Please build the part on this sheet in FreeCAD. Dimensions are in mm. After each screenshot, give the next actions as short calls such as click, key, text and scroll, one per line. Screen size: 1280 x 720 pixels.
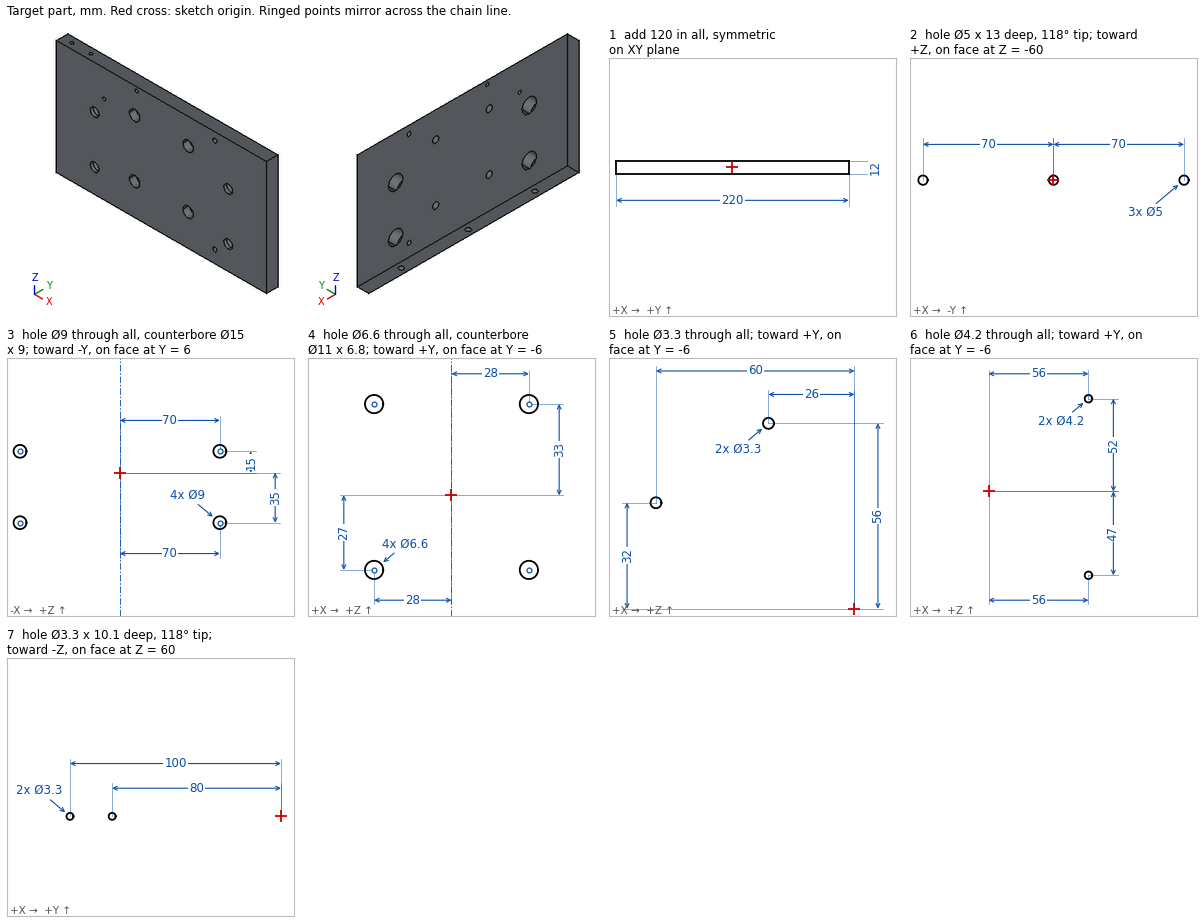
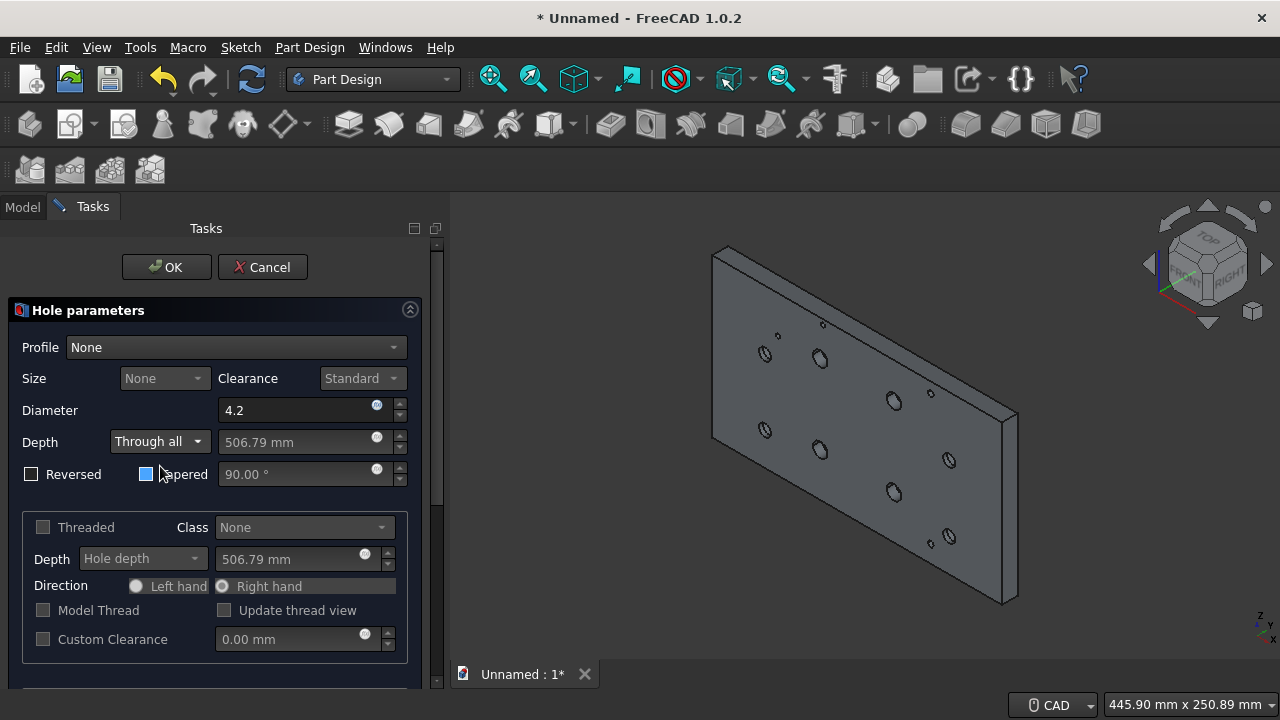
click(167, 267)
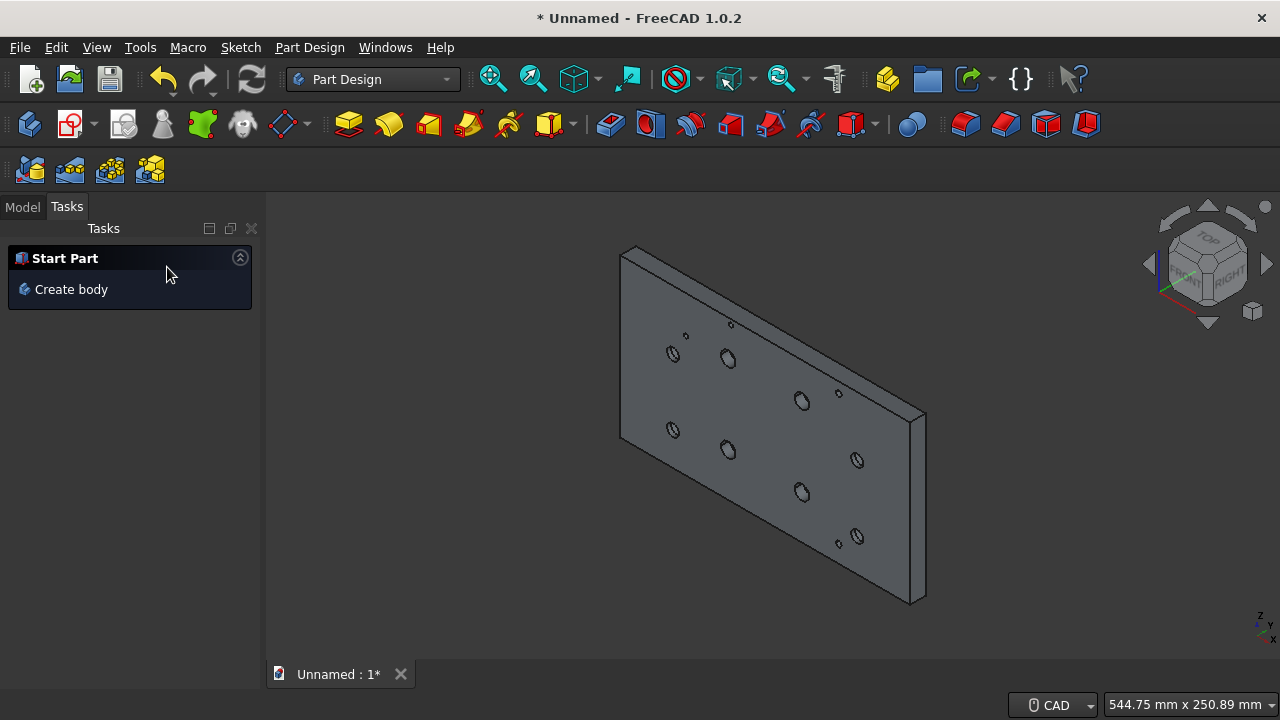
click(899, 404)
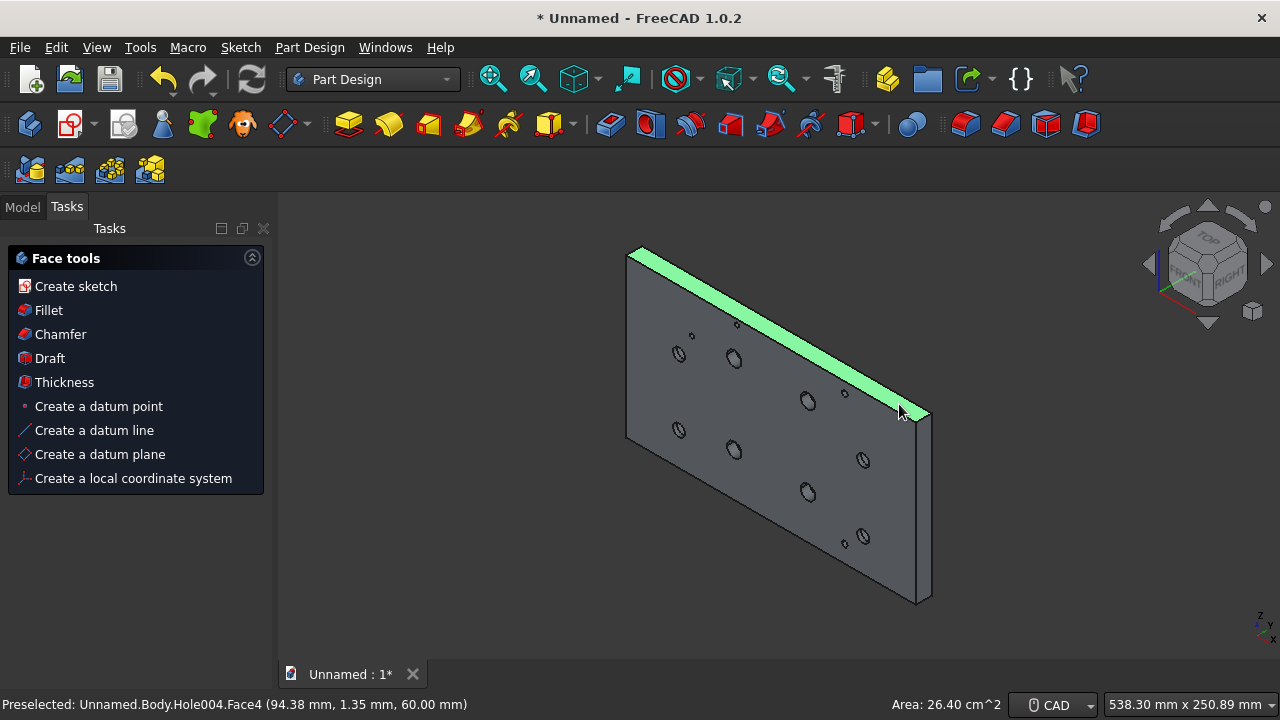
click(70, 124)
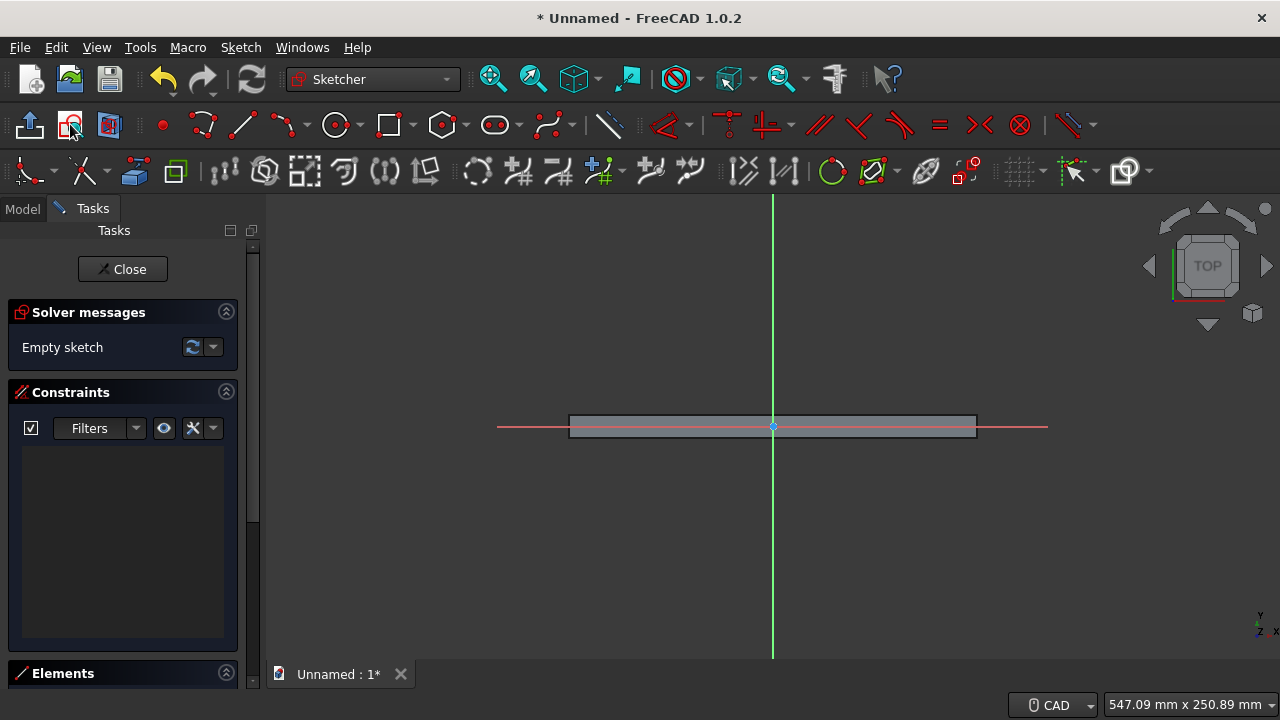
scroll(598, 426, up, 13)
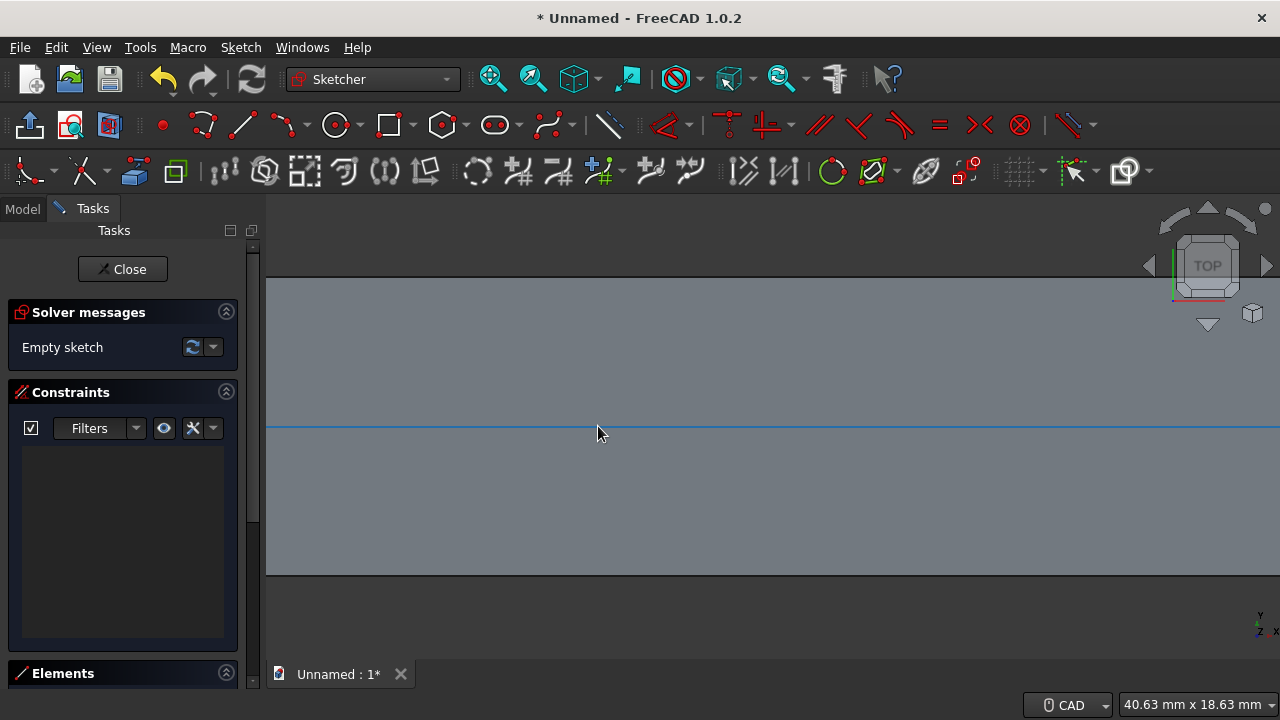
click(336, 126)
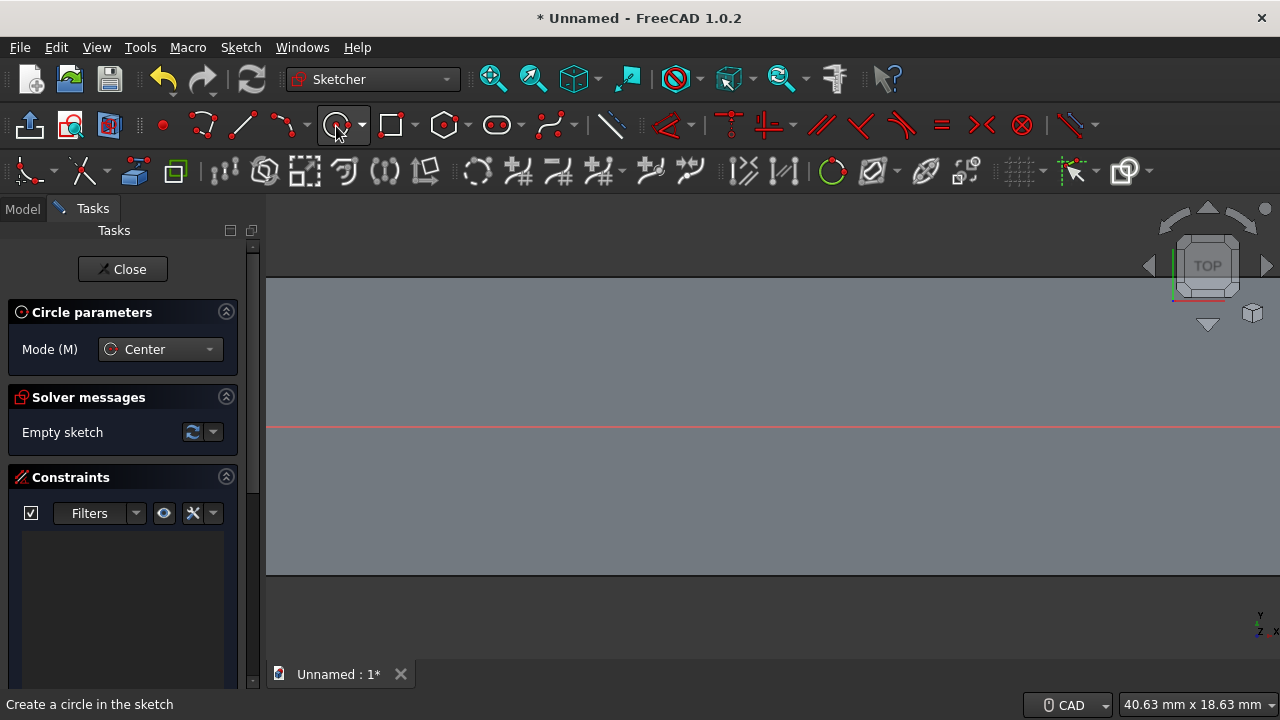
click(455, 426)
move(484, 397)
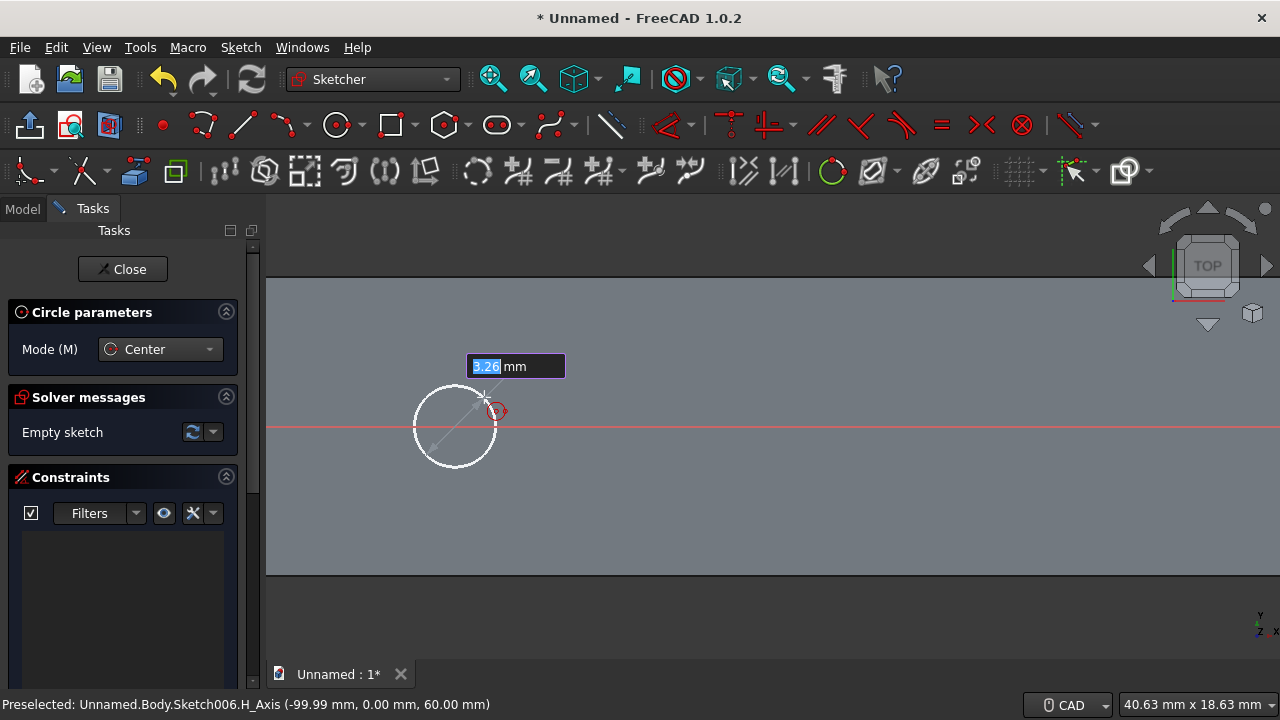
text(3.3)
key(Return)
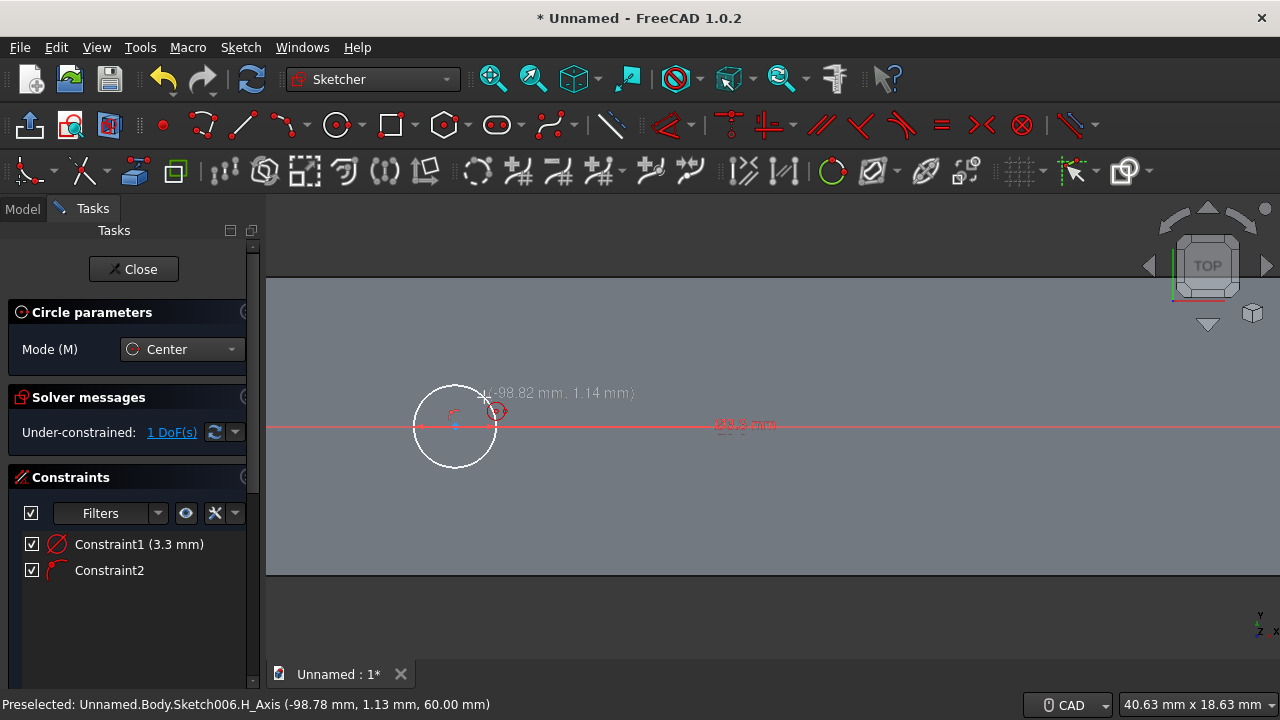
click(954, 426)
move(983, 397)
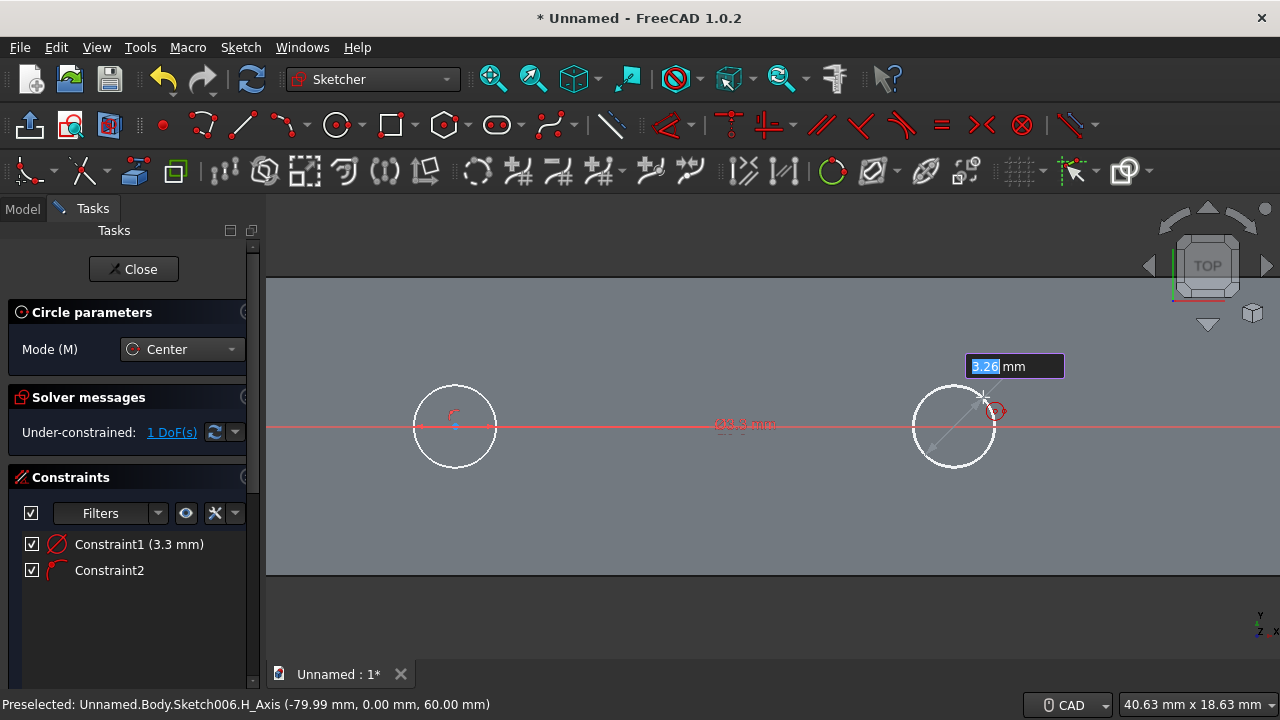
text(3.3)
key(Return)
key(Escape)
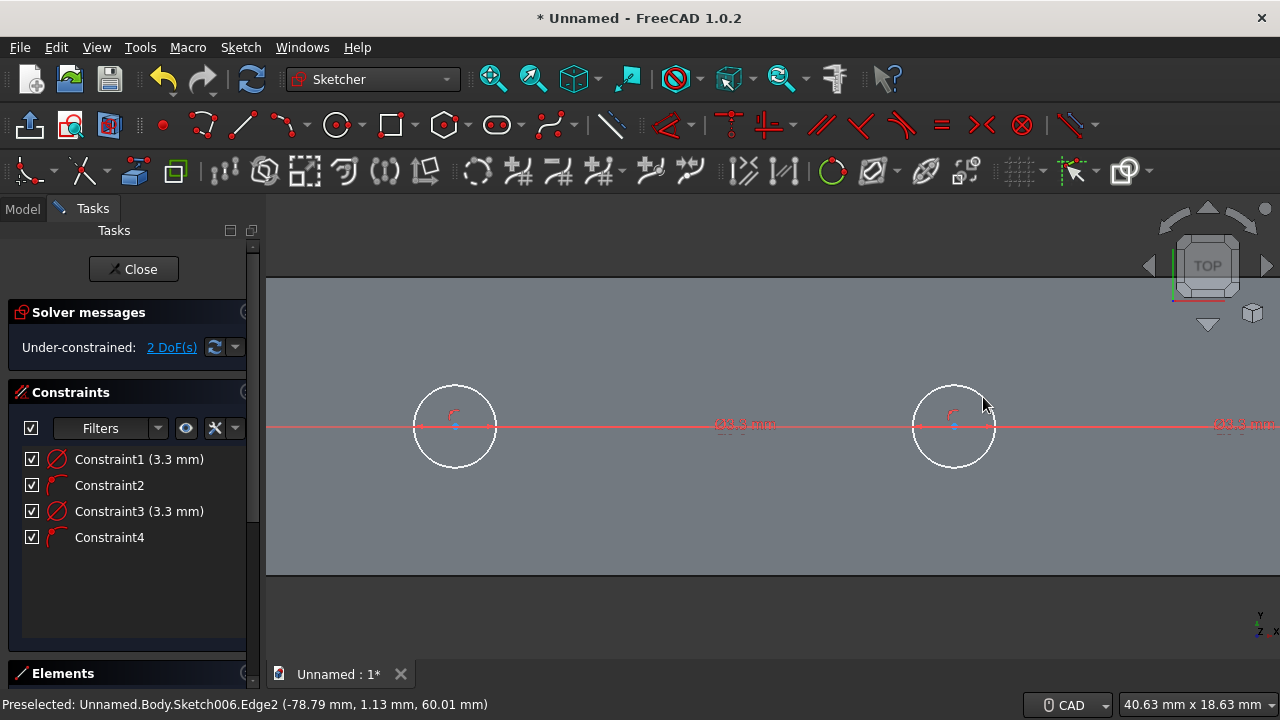
click(666, 126)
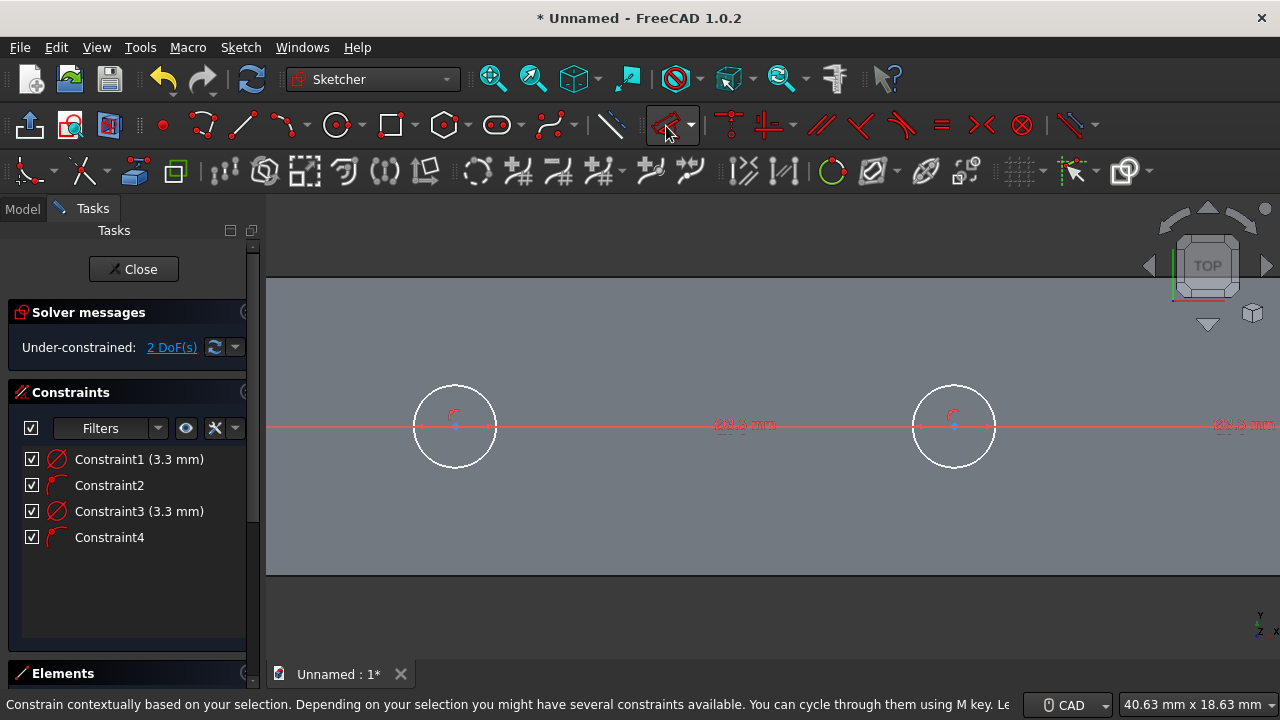
click(954, 426)
click(1034, 460)